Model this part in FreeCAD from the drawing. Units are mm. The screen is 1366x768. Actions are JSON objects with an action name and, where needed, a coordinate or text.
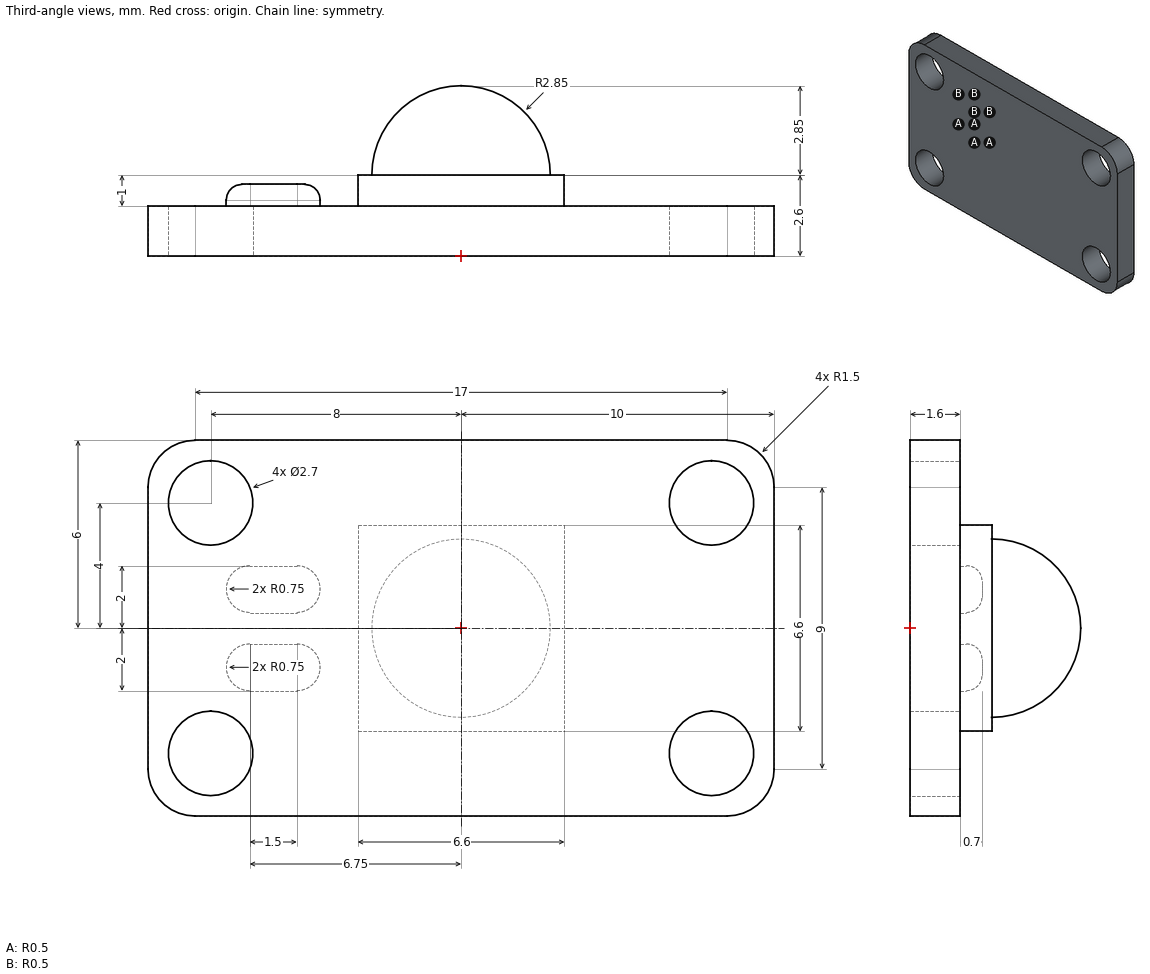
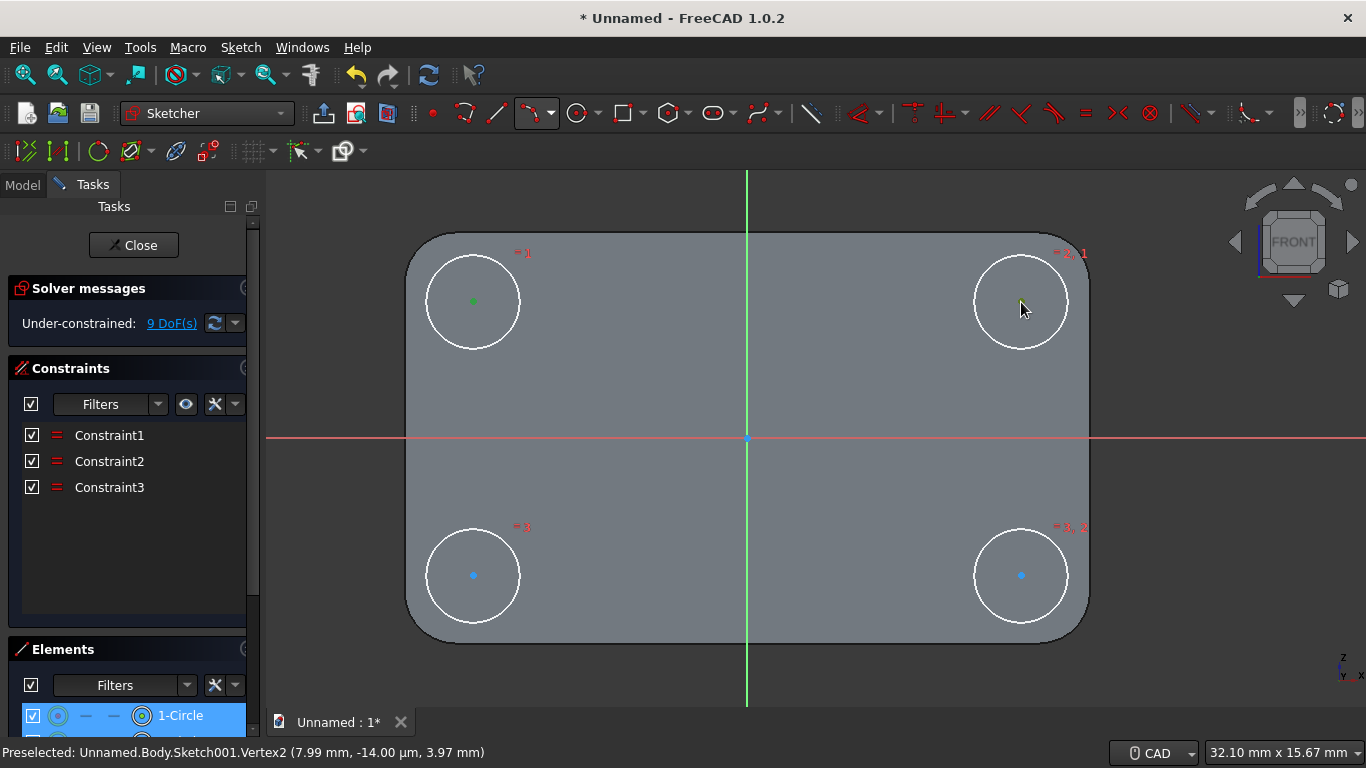
{"action": "left_click", "coordinate": [747, 645]}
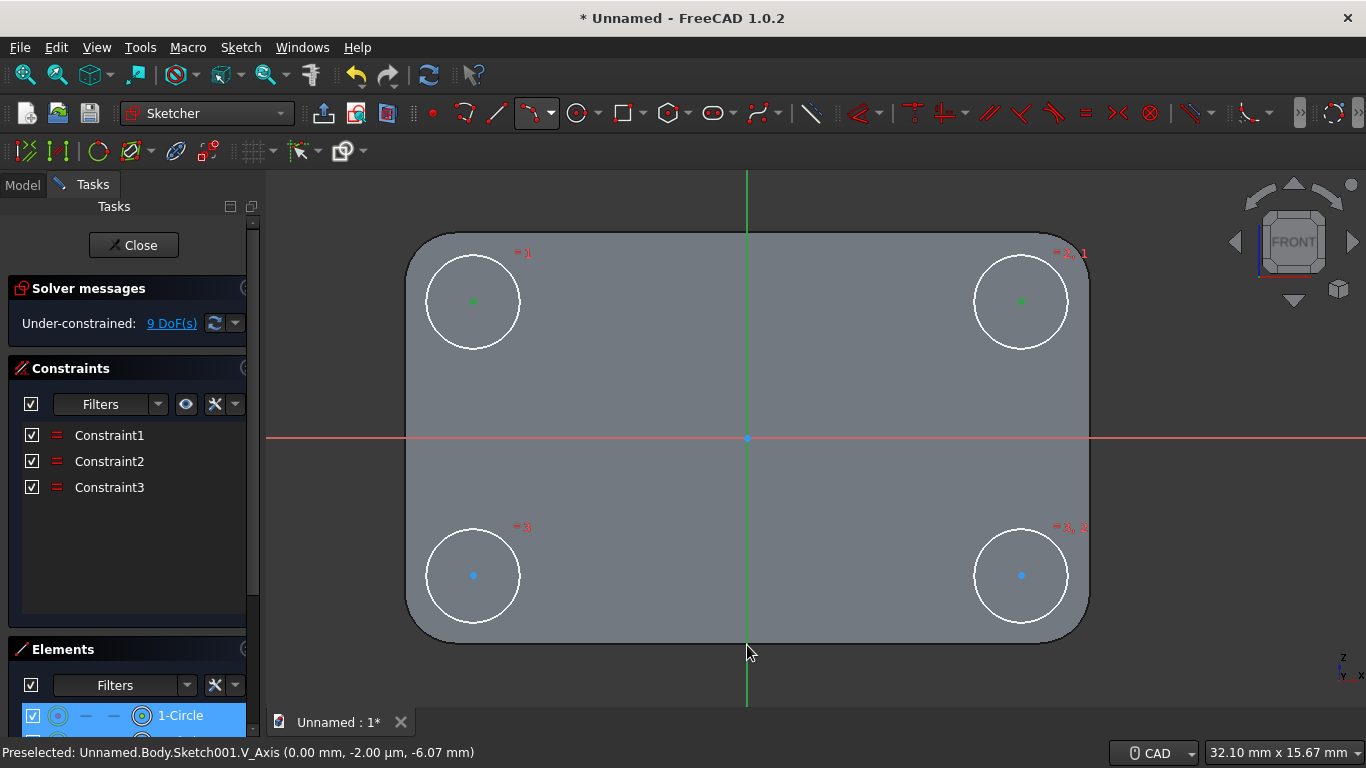
{"action": "left_click", "coordinate": [1118, 114]}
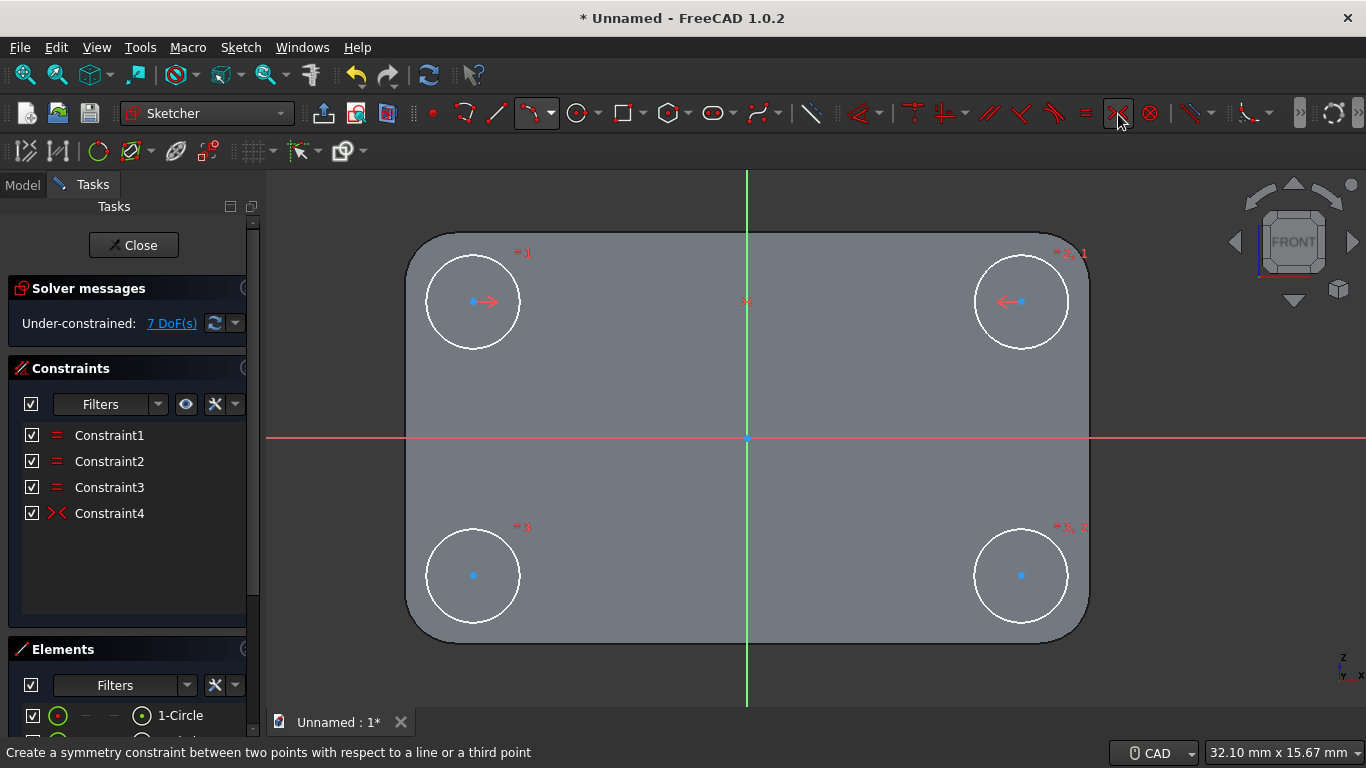
{"action": "left_click", "coordinate": [1022, 302]}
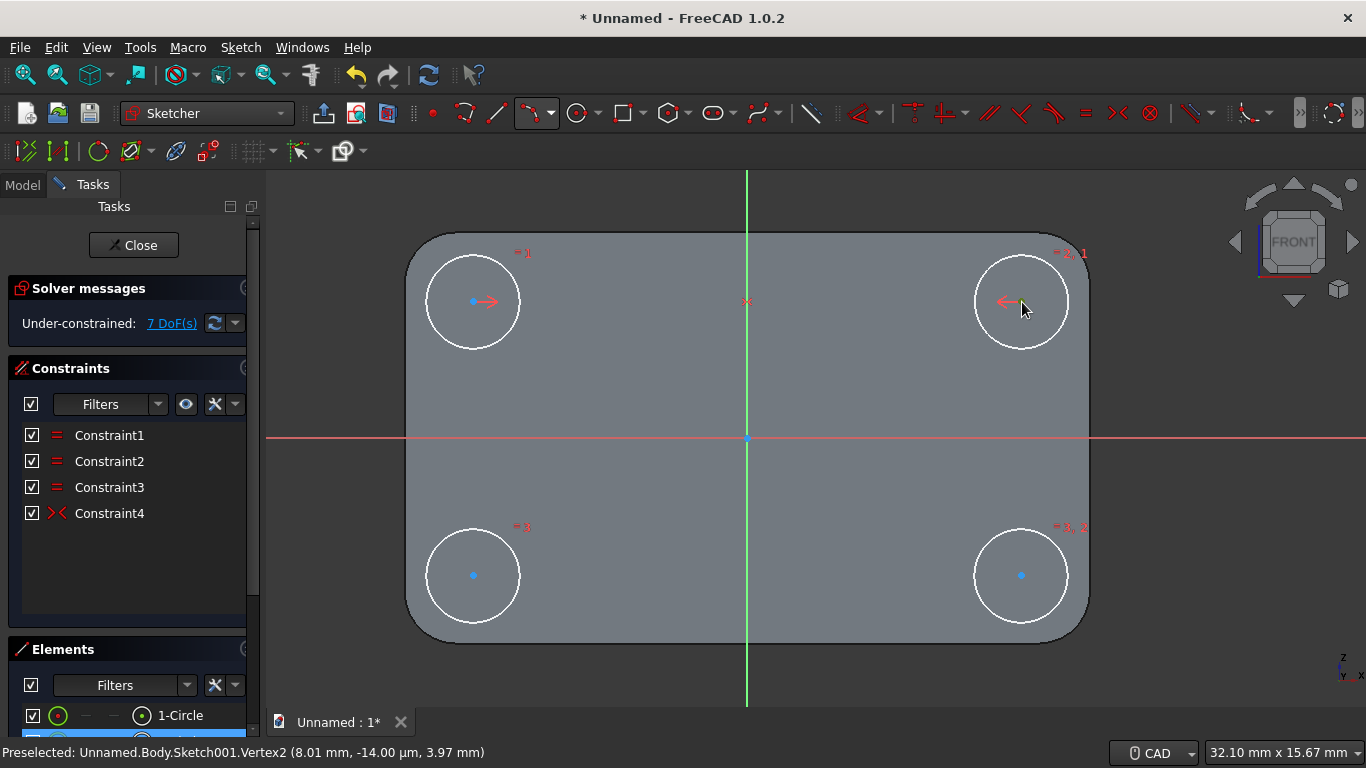
{"action": "left_click", "coordinate": [1021, 576]}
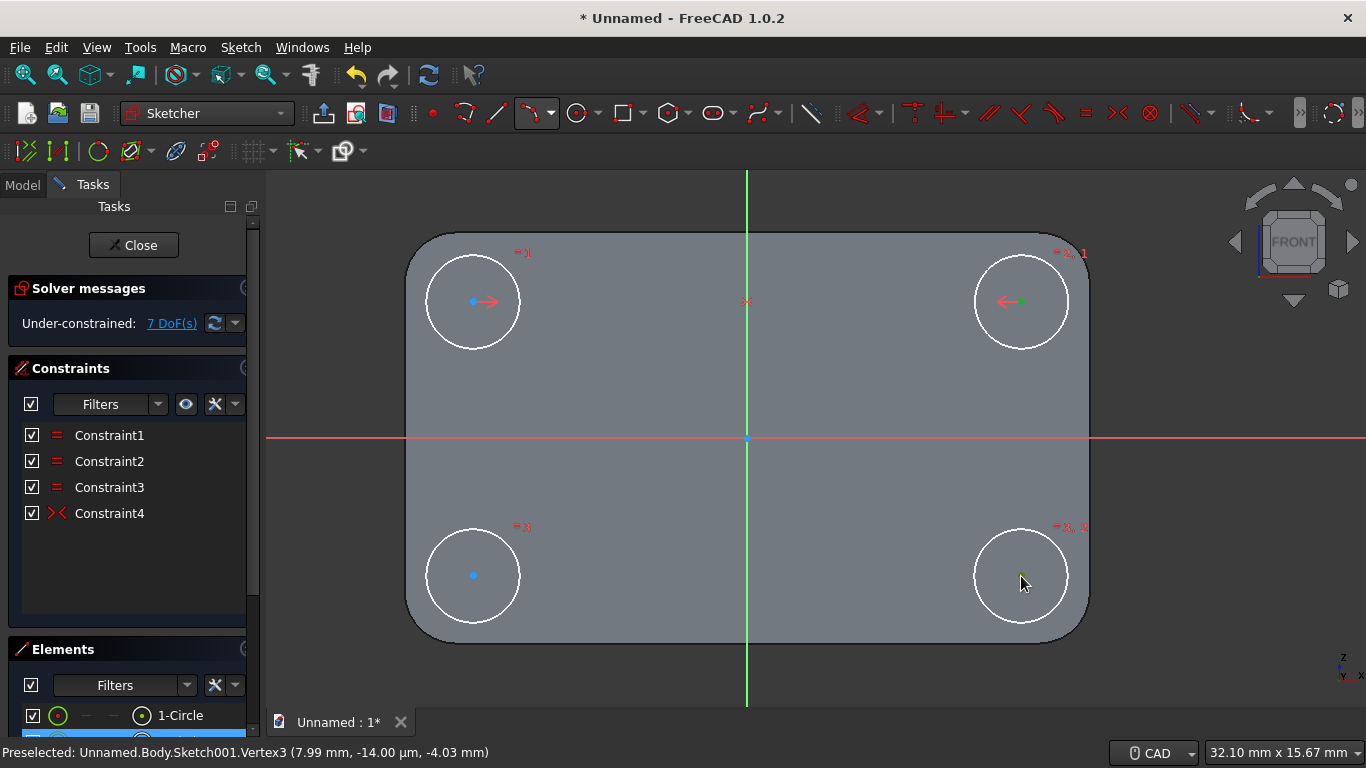
{"action": "left_click", "coordinate": [359, 438]}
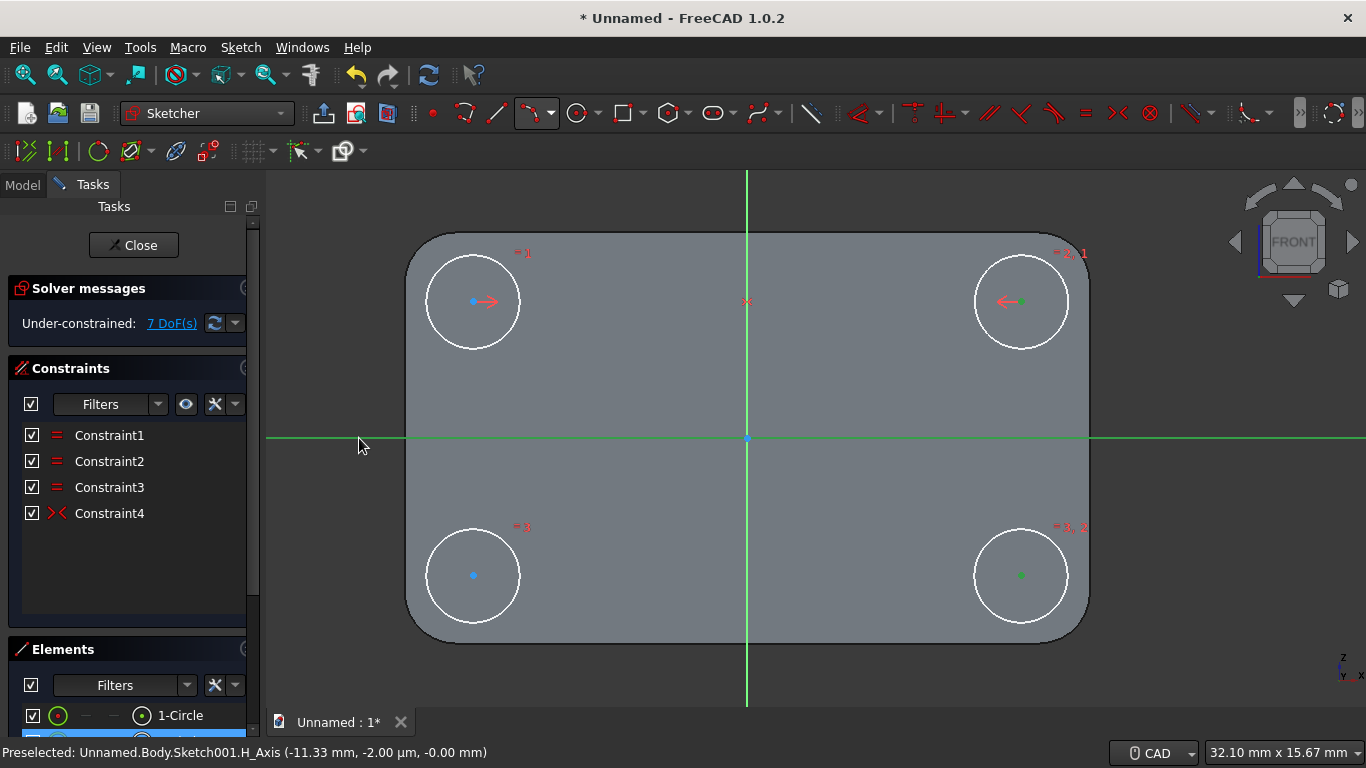
{"action": "left_click", "coordinate": [1118, 114]}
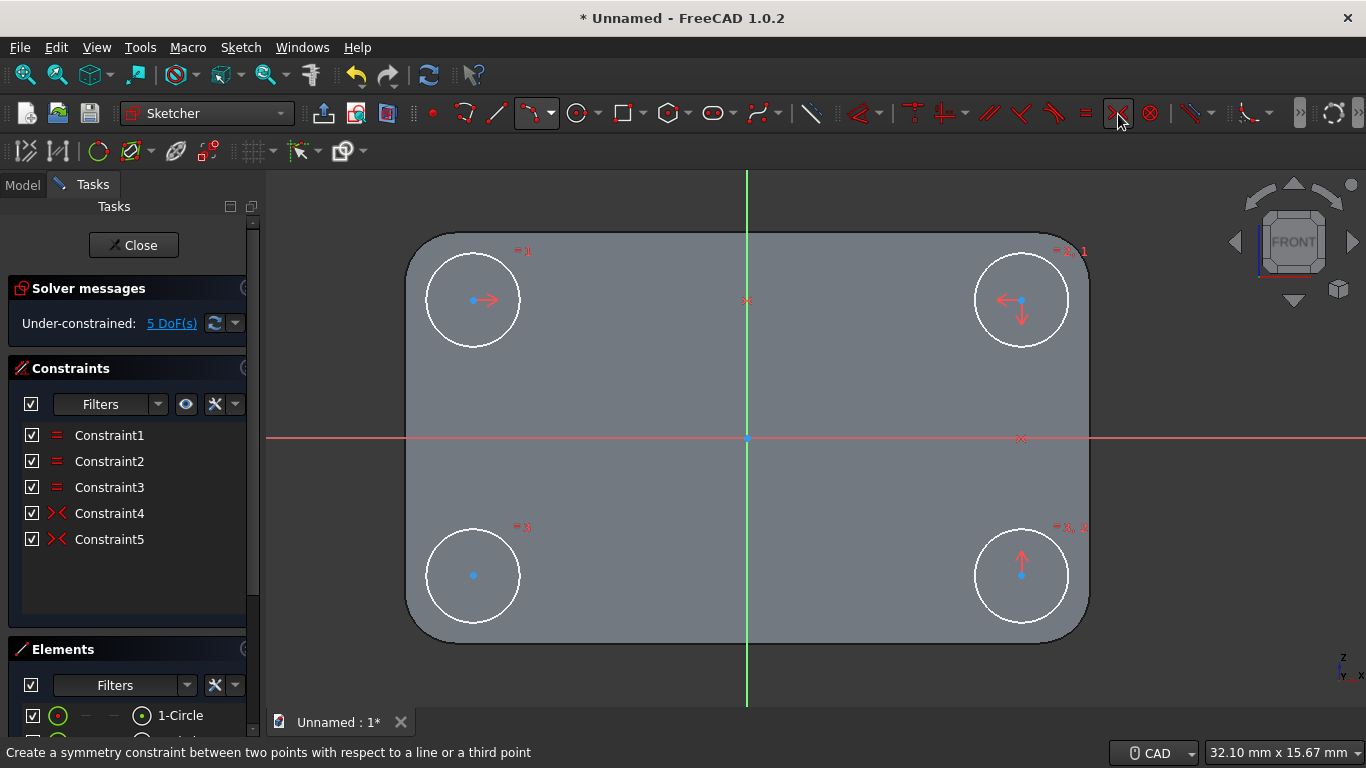
{"action": "left_click", "coordinate": [473, 300]}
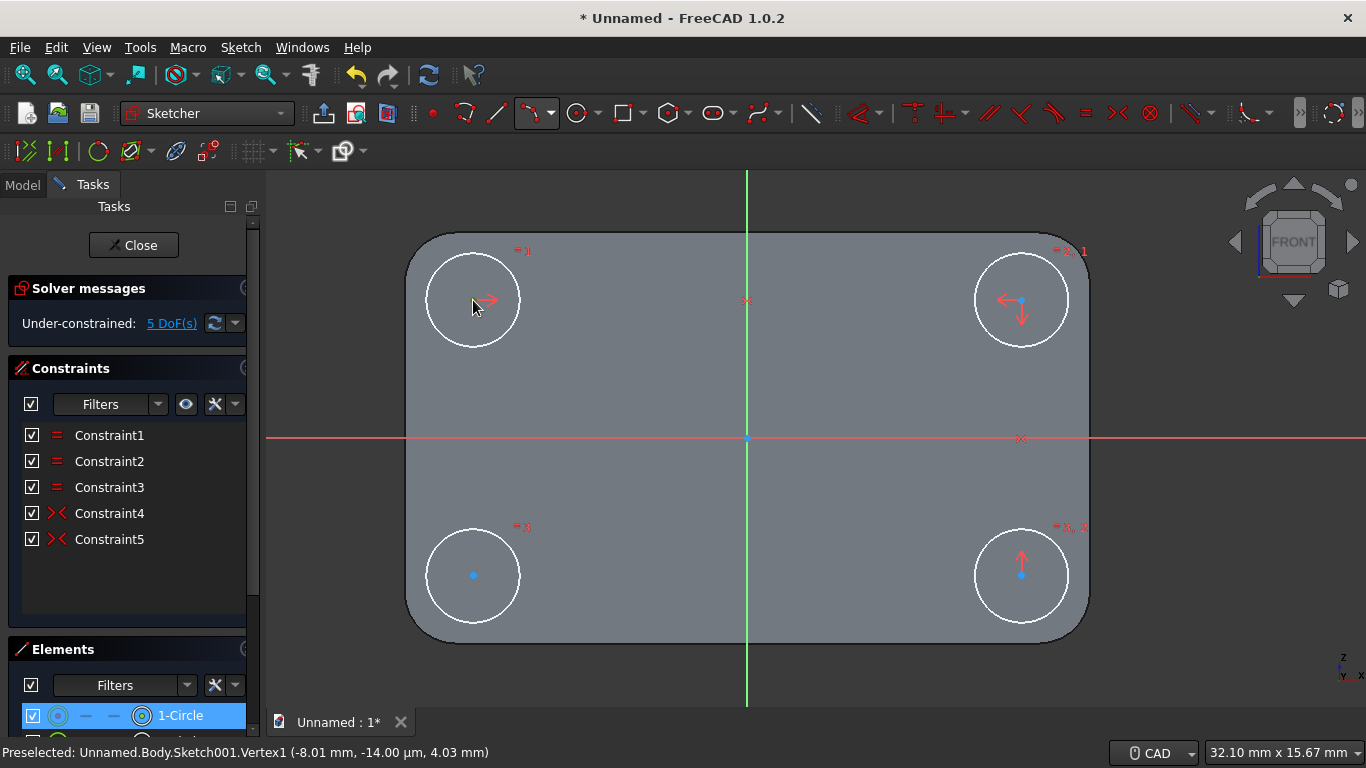
{"action": "left_click", "coordinate": [473, 576]}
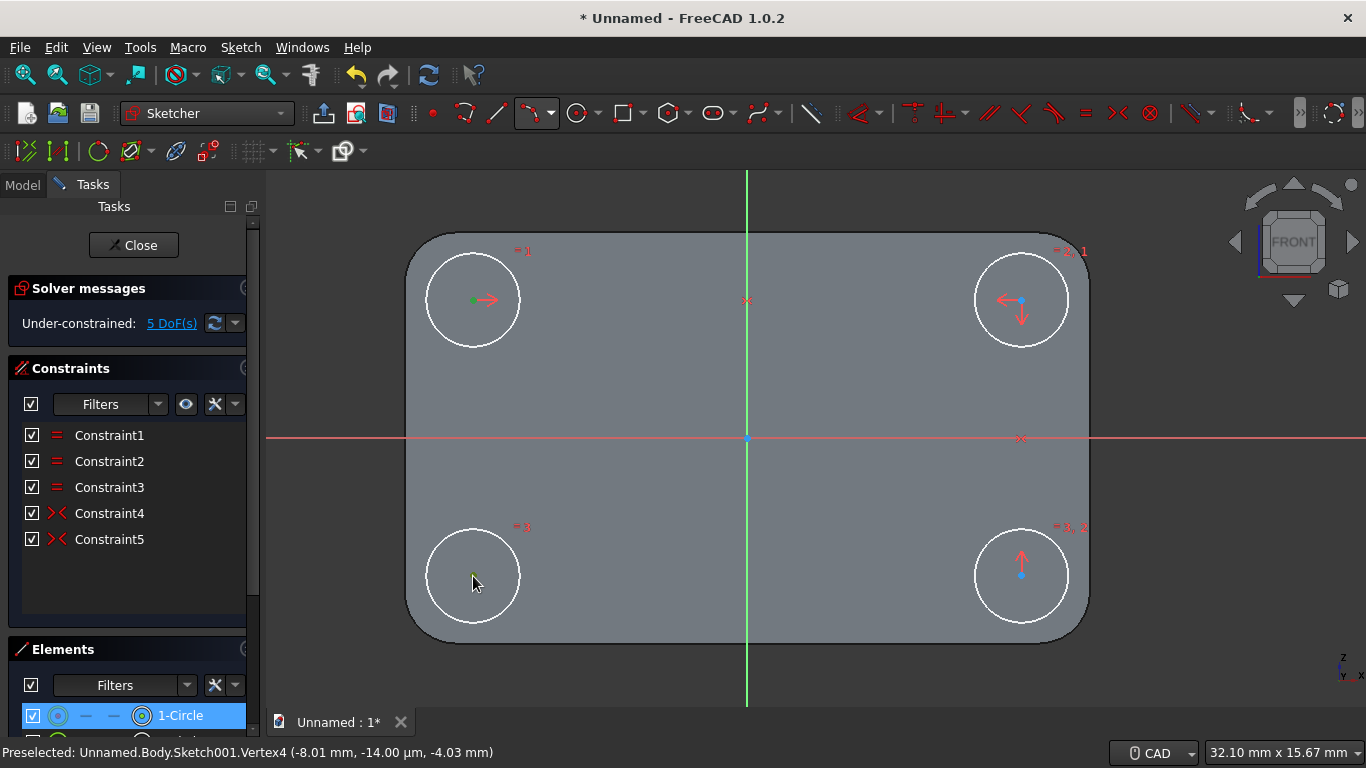
{"action": "left_click", "coordinate": [359, 438]}